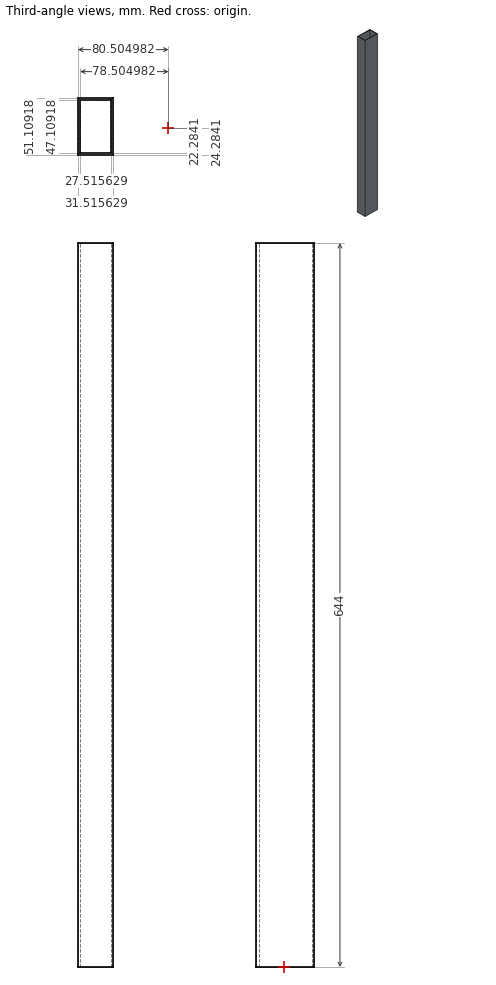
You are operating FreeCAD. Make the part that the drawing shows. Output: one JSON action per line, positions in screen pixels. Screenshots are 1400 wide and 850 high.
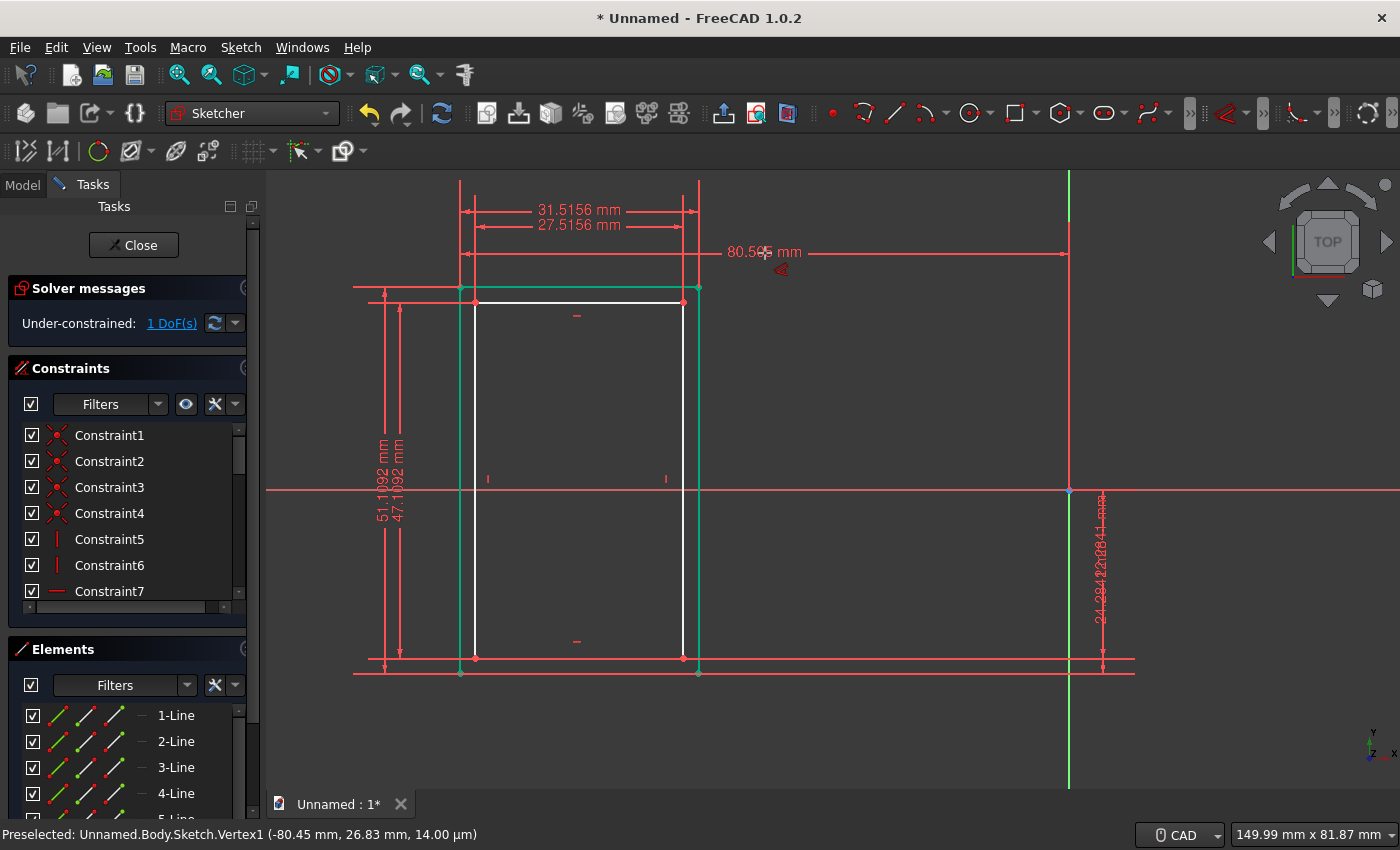
{"action": "left_click", "coordinate": [475, 302]}
{"action": "left_click", "coordinate": [636, 268]}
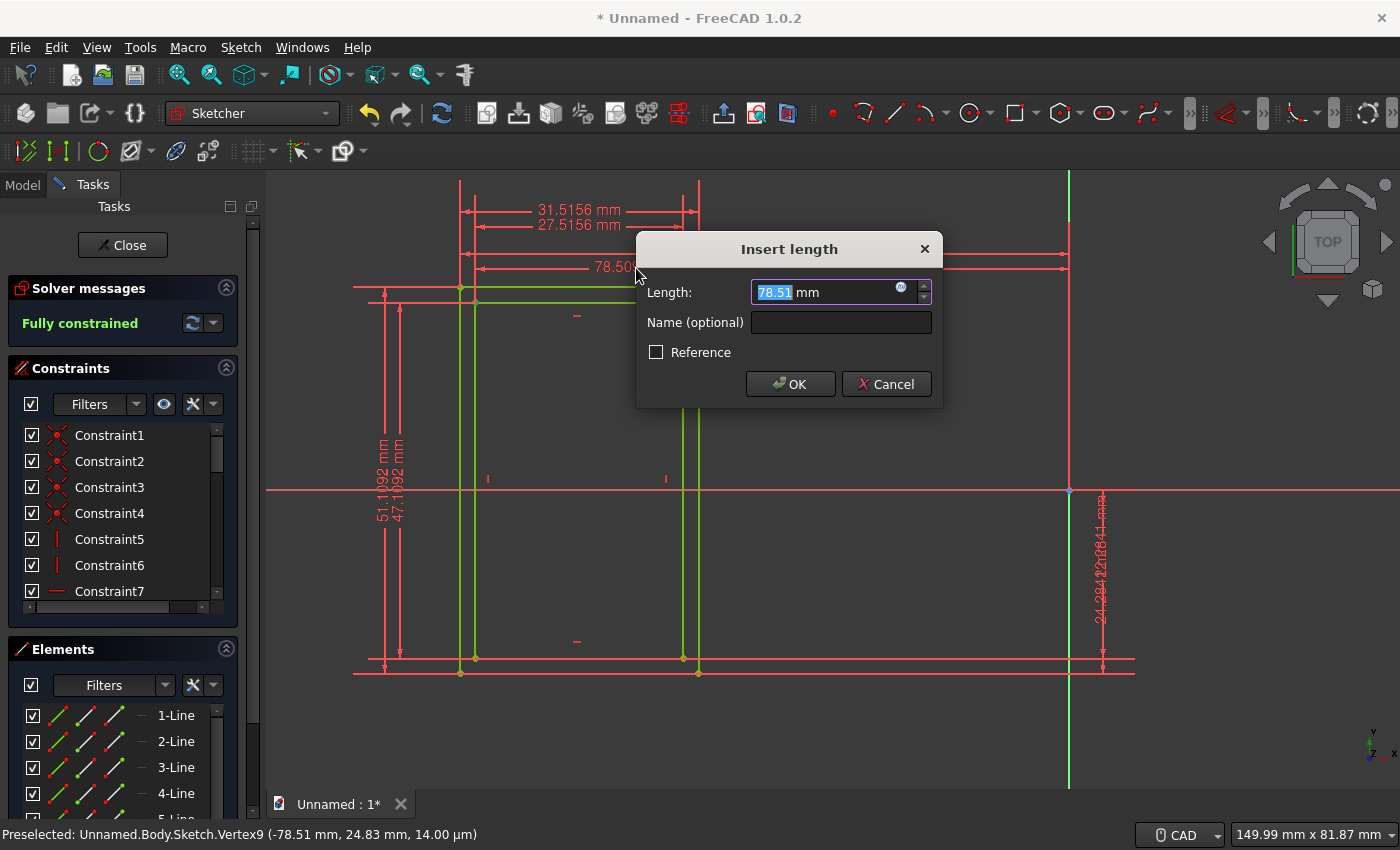
{"action": "type", "text": "78.504982"}
{"action": "key", "text": "Return"}
{"action": "key", "text": "Escape"}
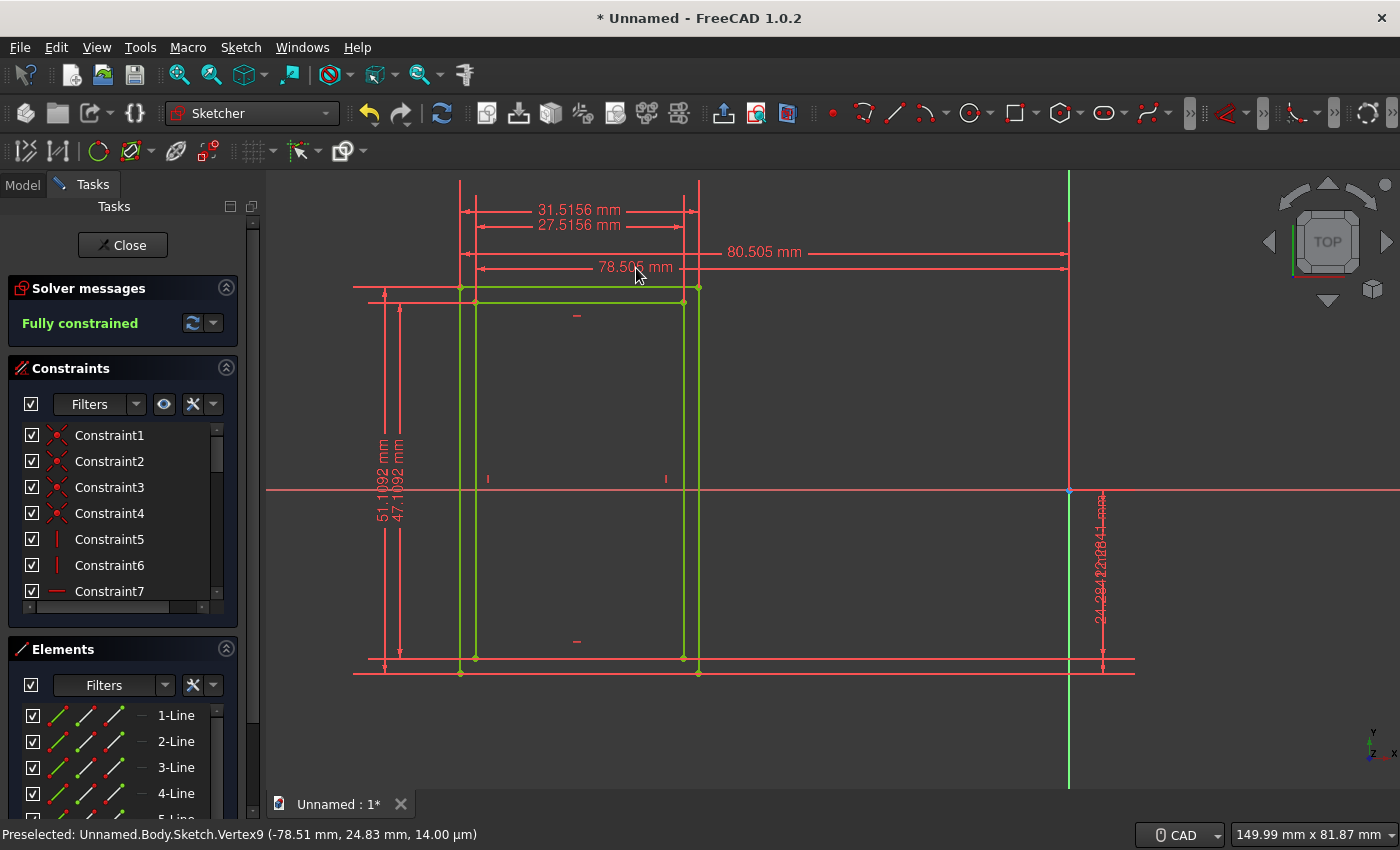
{"action": "left_click", "coordinate": [123, 245]}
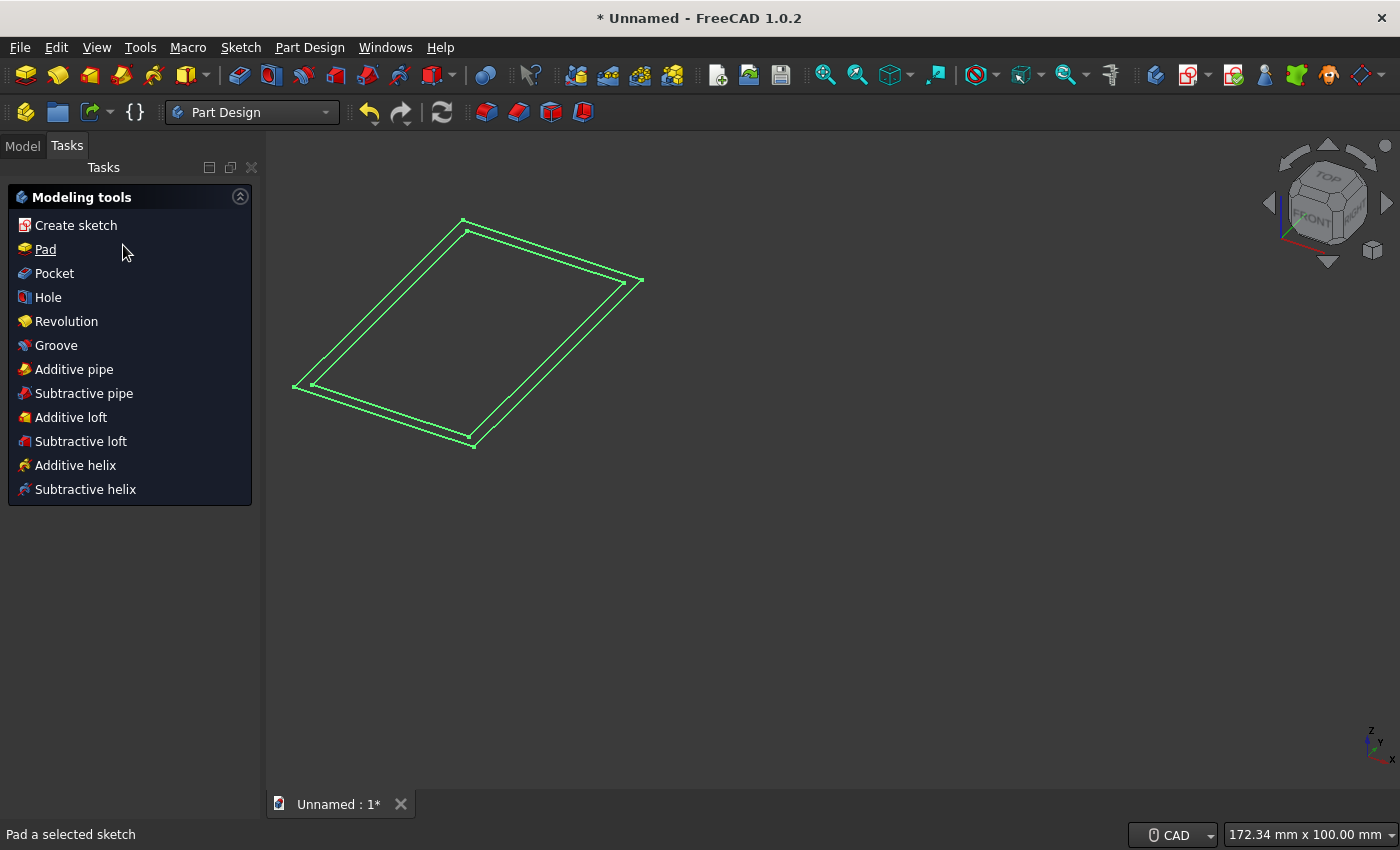
{"action": "left_click", "coordinate": [26, 76]}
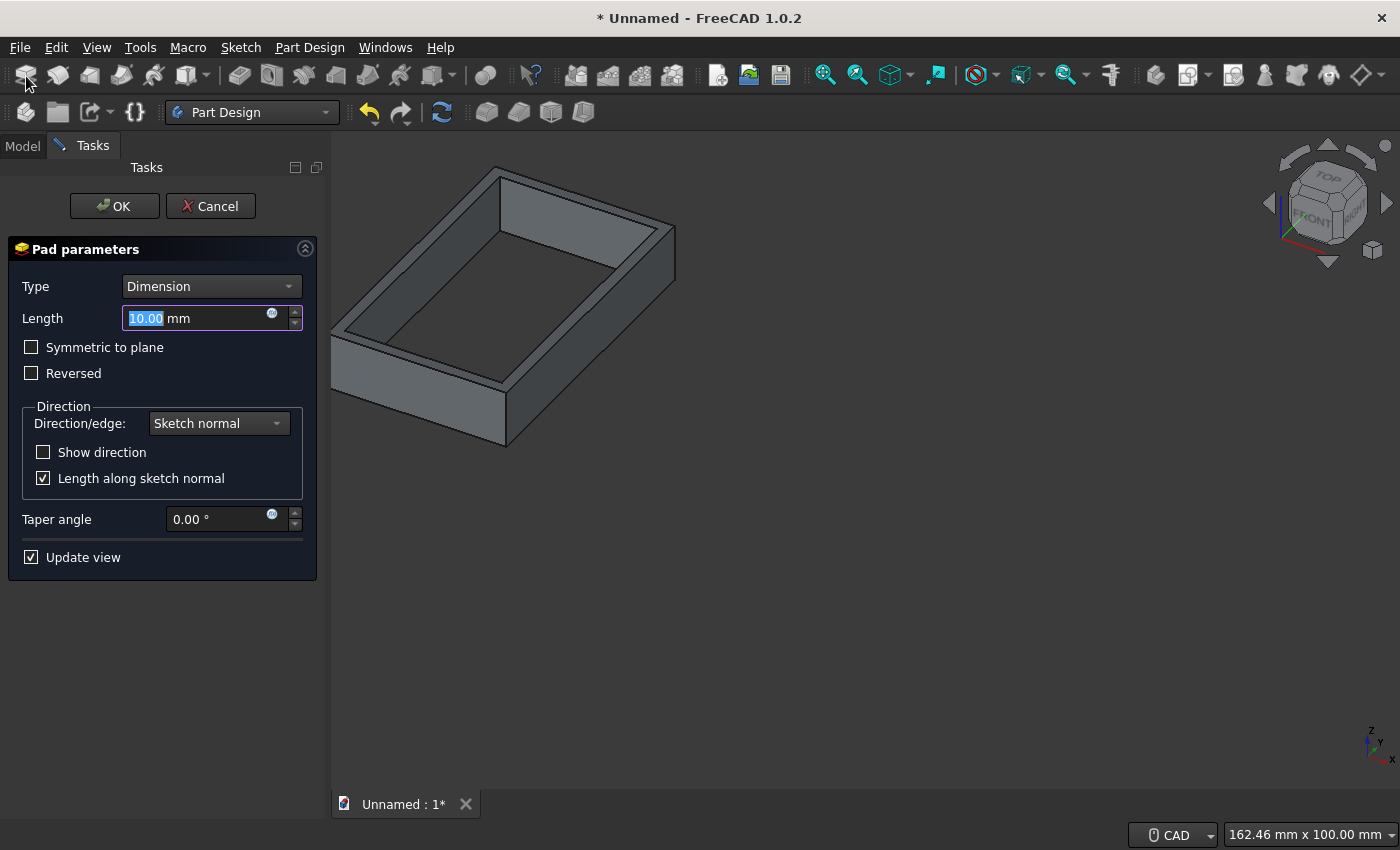
{"action": "type", "text": "644"}
{"action": "key", "text": "Tab"}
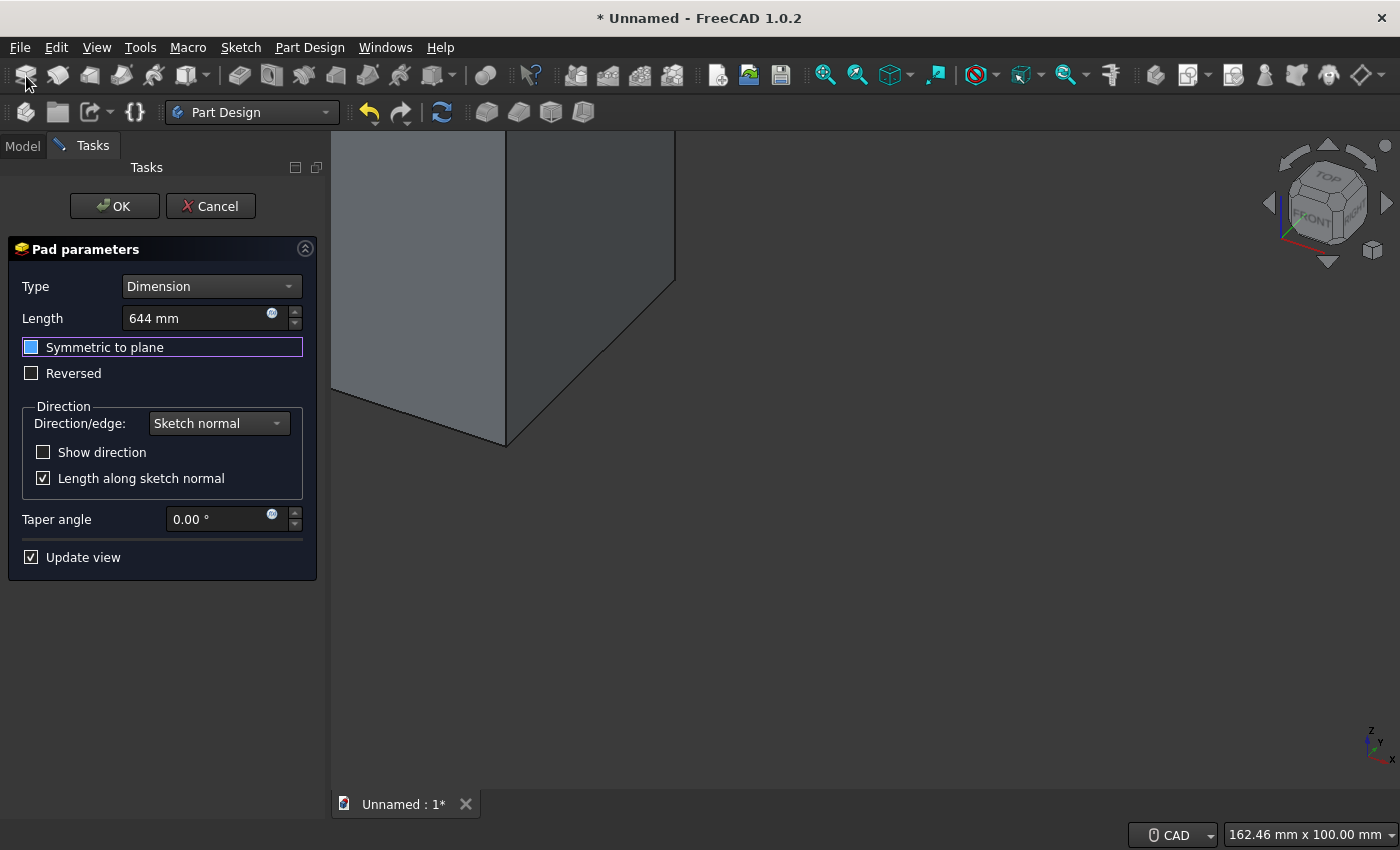
{"action": "left_click", "coordinate": [115, 206]}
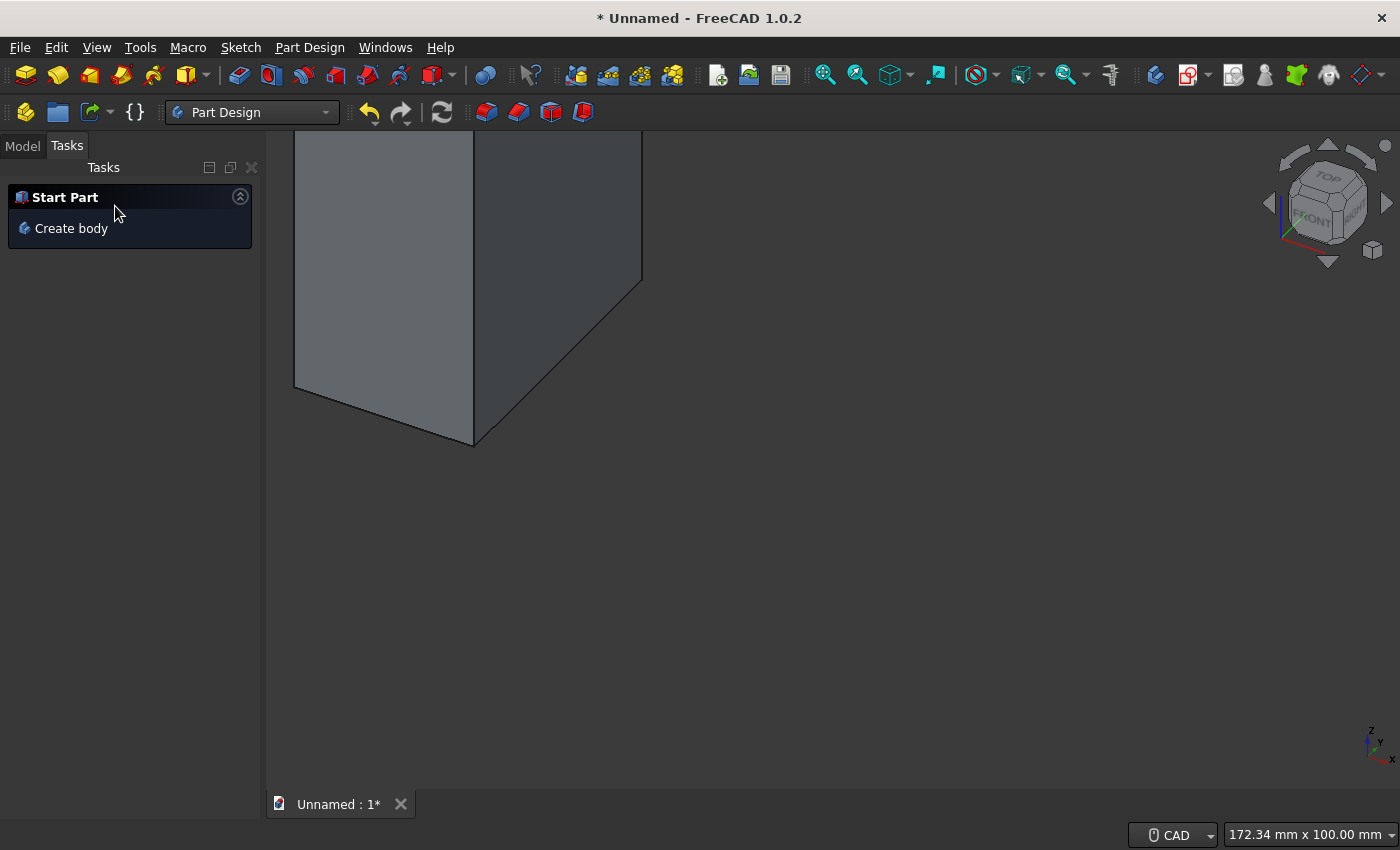
{"action": "key", "text": "0"}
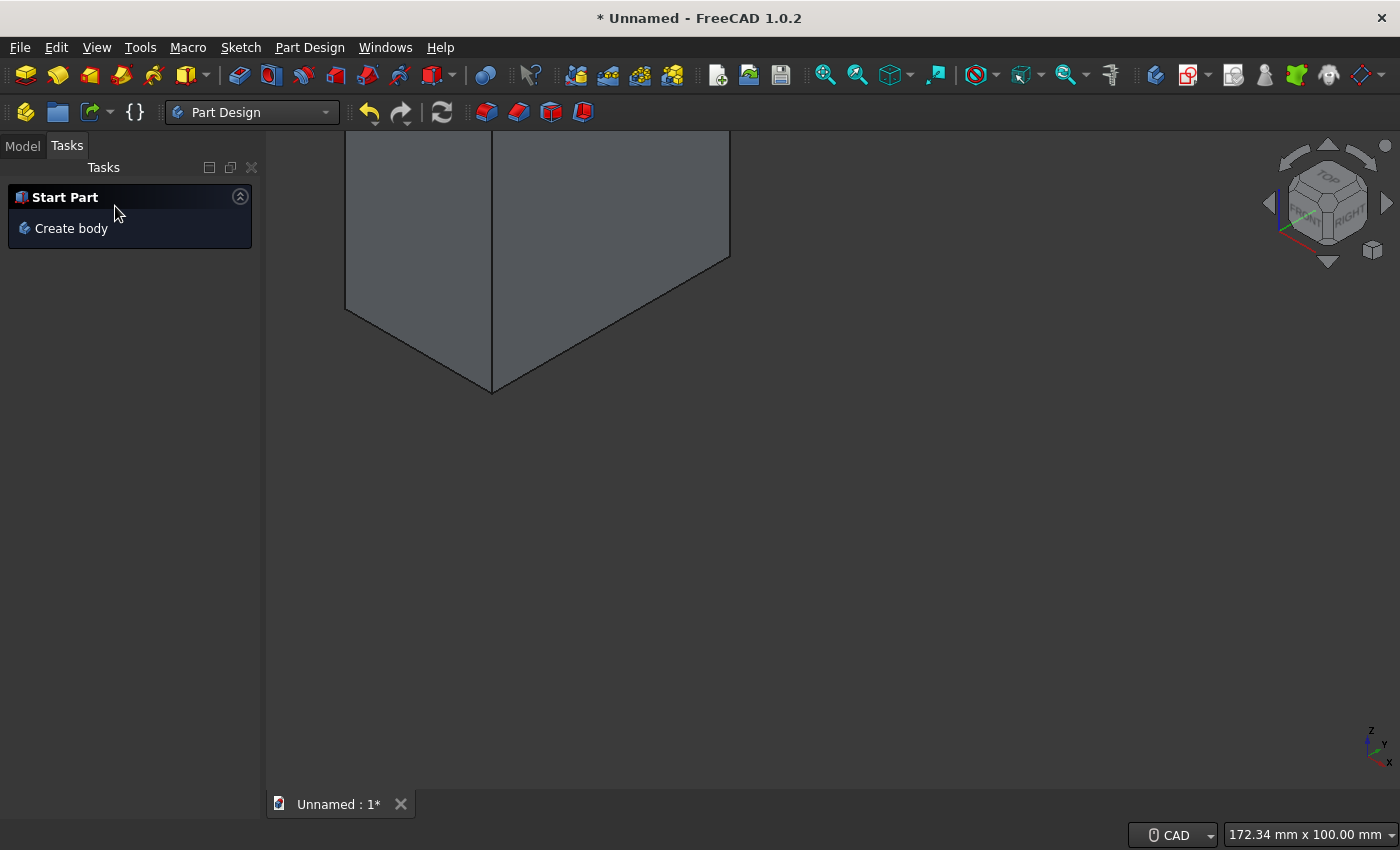
{"action": "key", "text": "v f"}